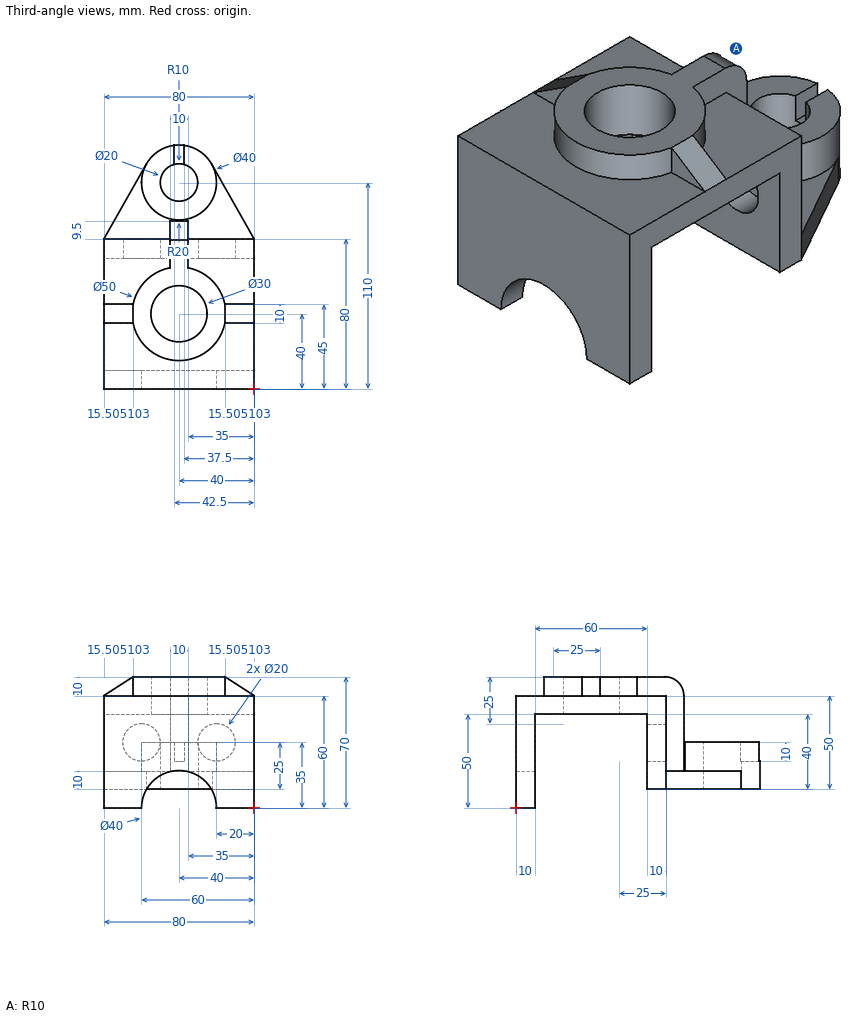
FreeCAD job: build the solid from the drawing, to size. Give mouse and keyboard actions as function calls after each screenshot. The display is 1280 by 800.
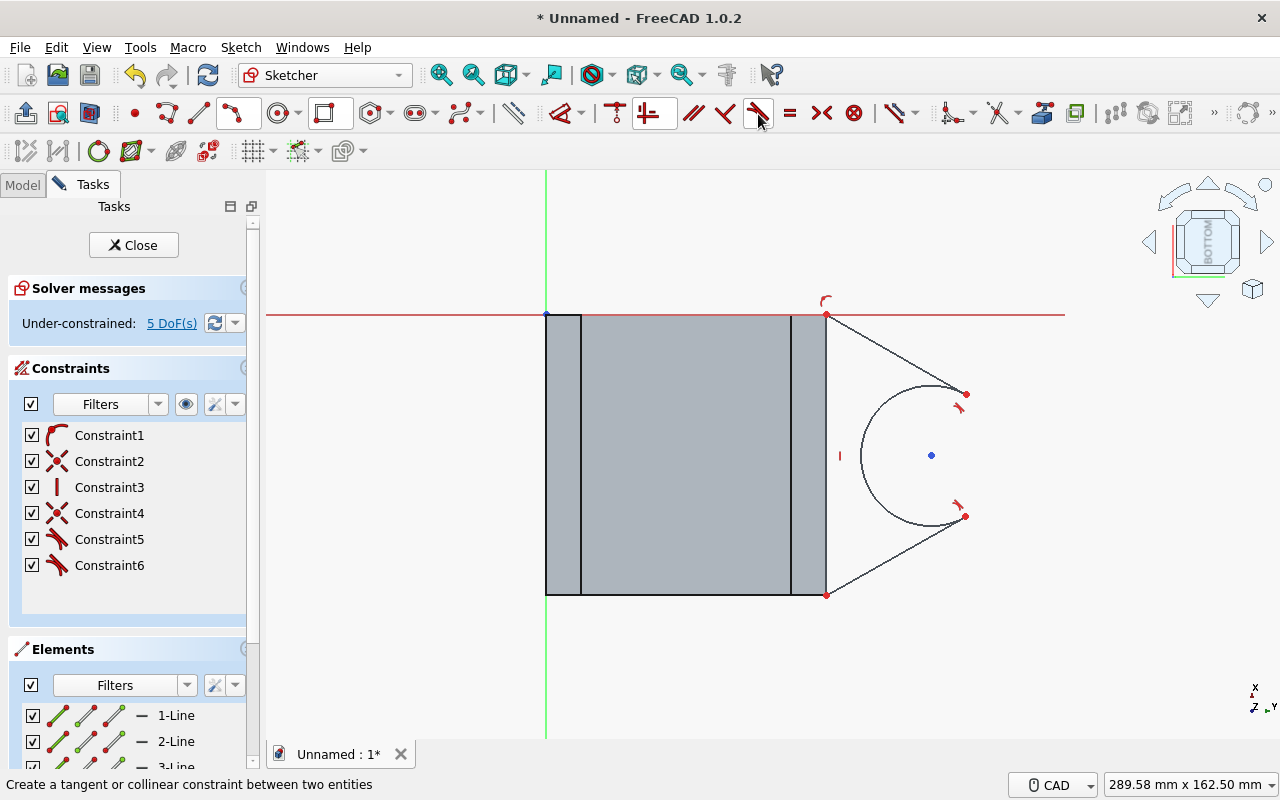
click(560, 114)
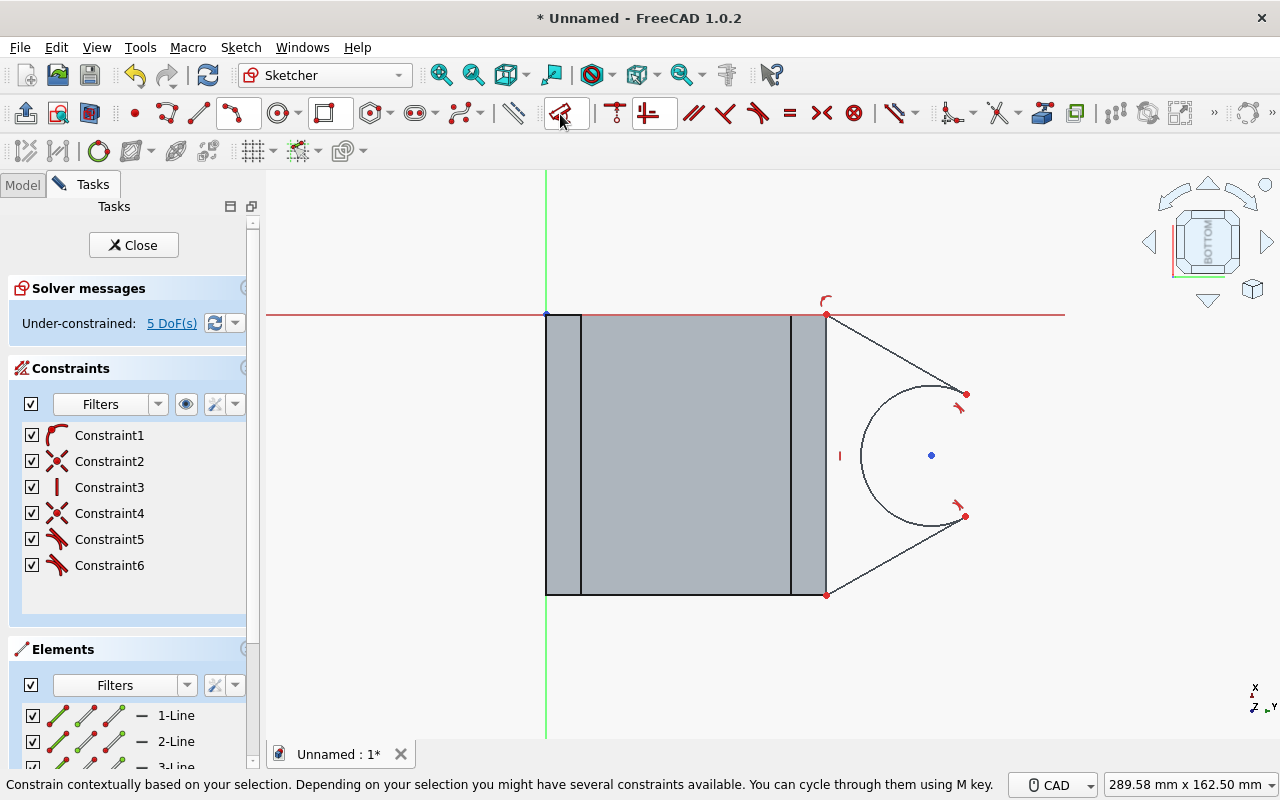
click(884, 404)
click(862, 380)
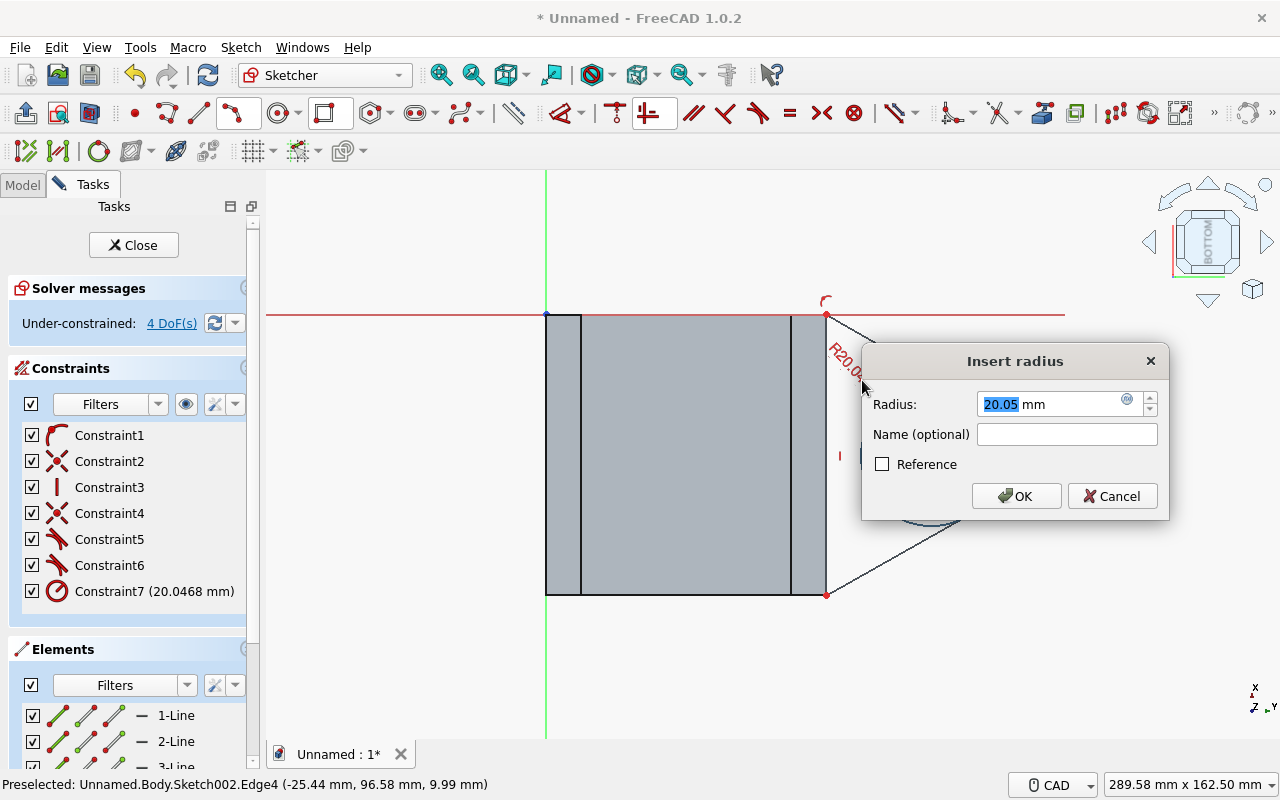
text(20)
key(Return)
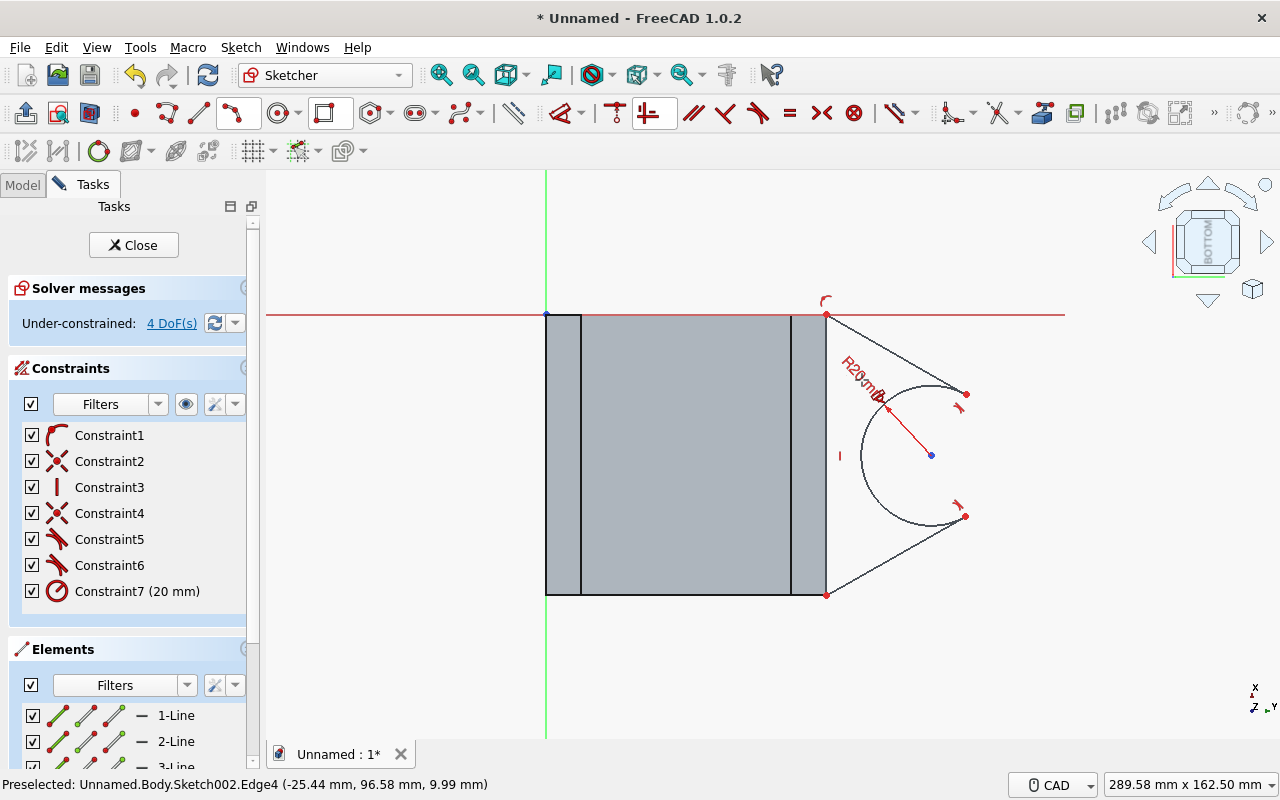
click(826, 399)
click(860, 520)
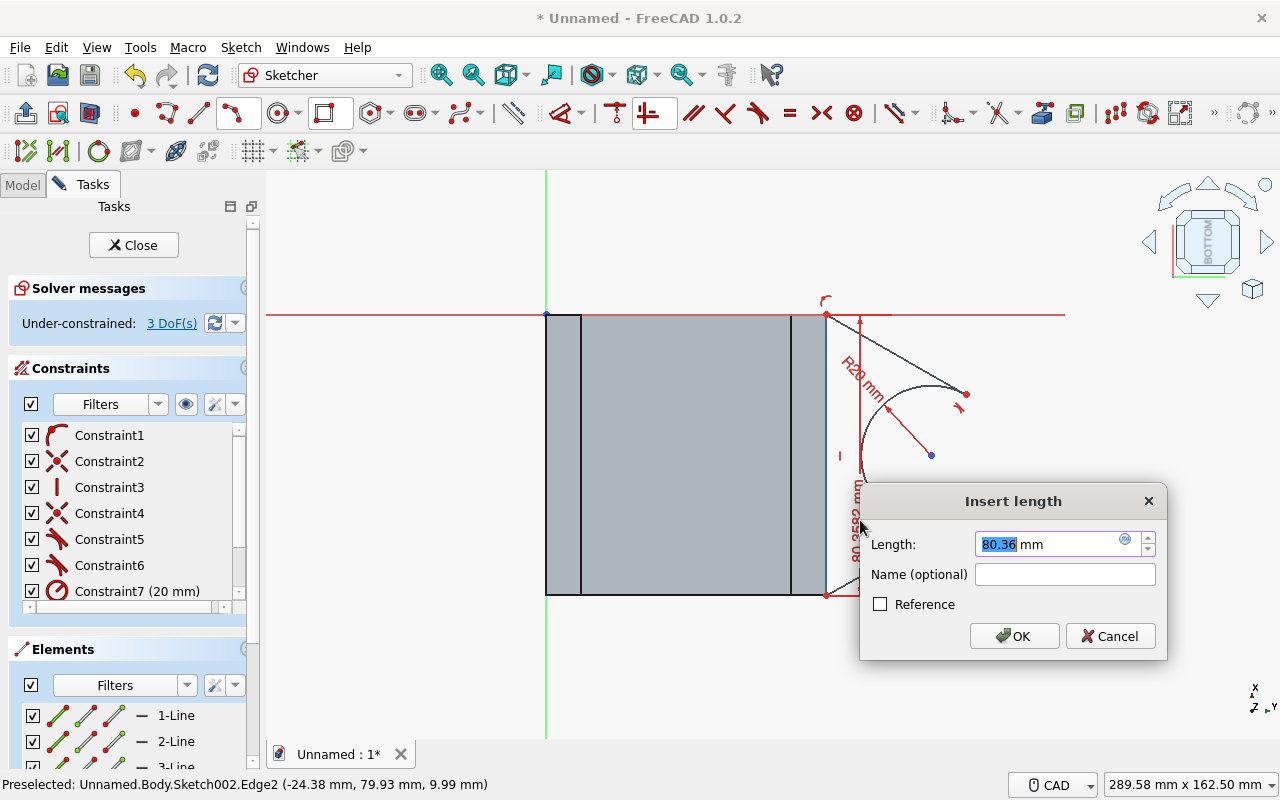
text(80)
key(Return)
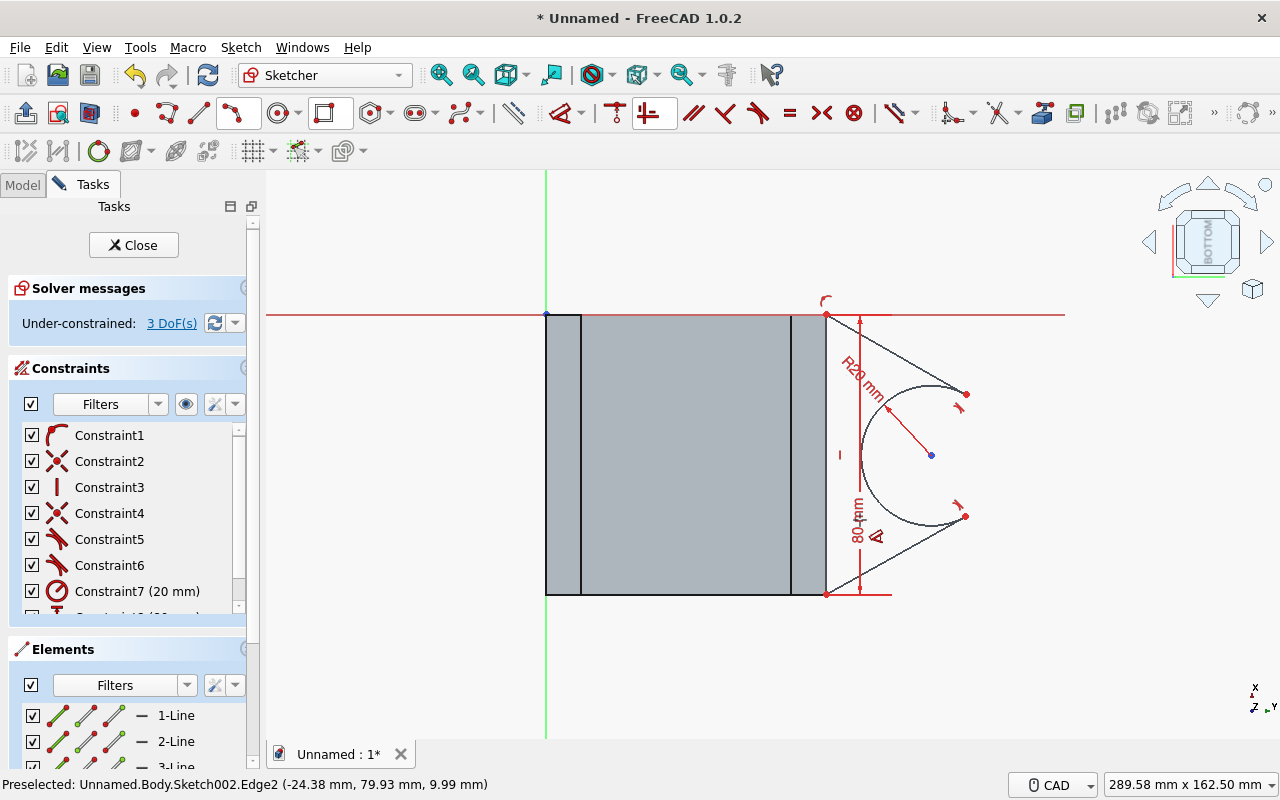
click(826, 315)
click(686, 281)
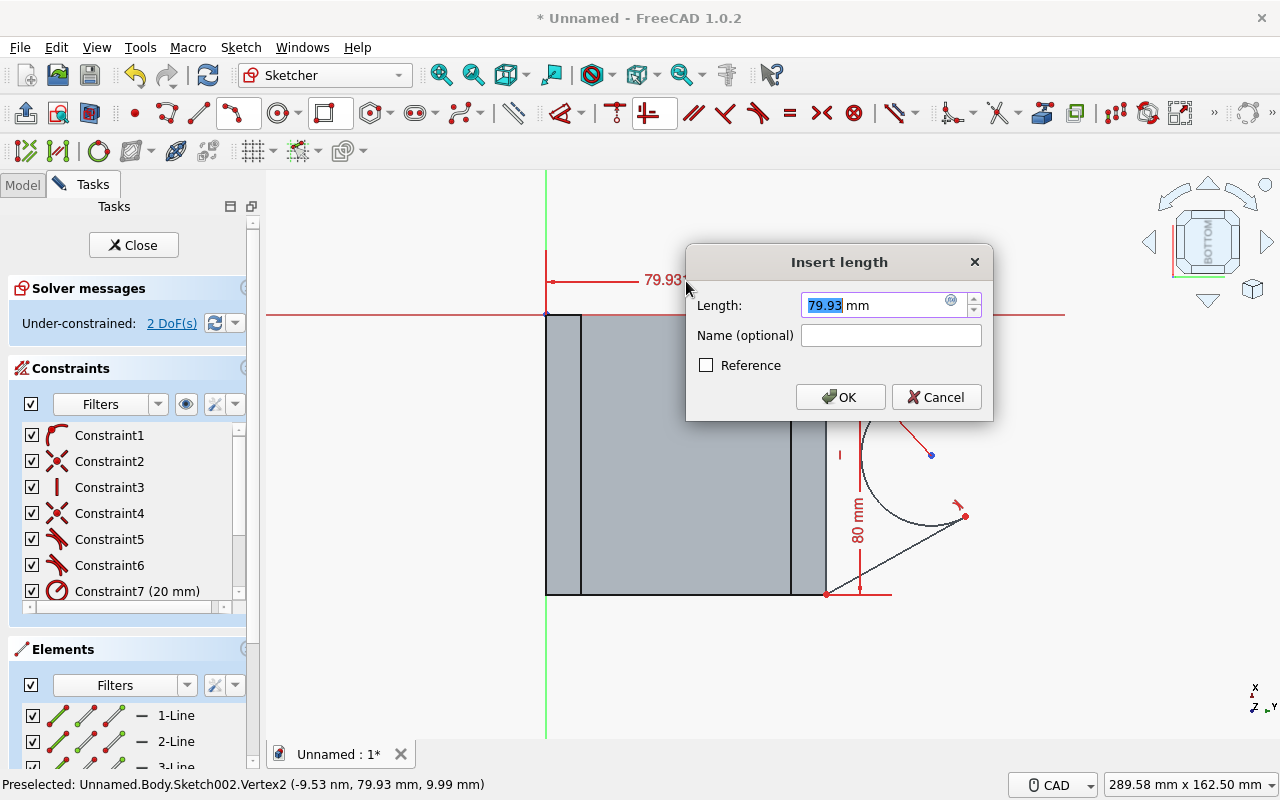
text(80)
key(Return)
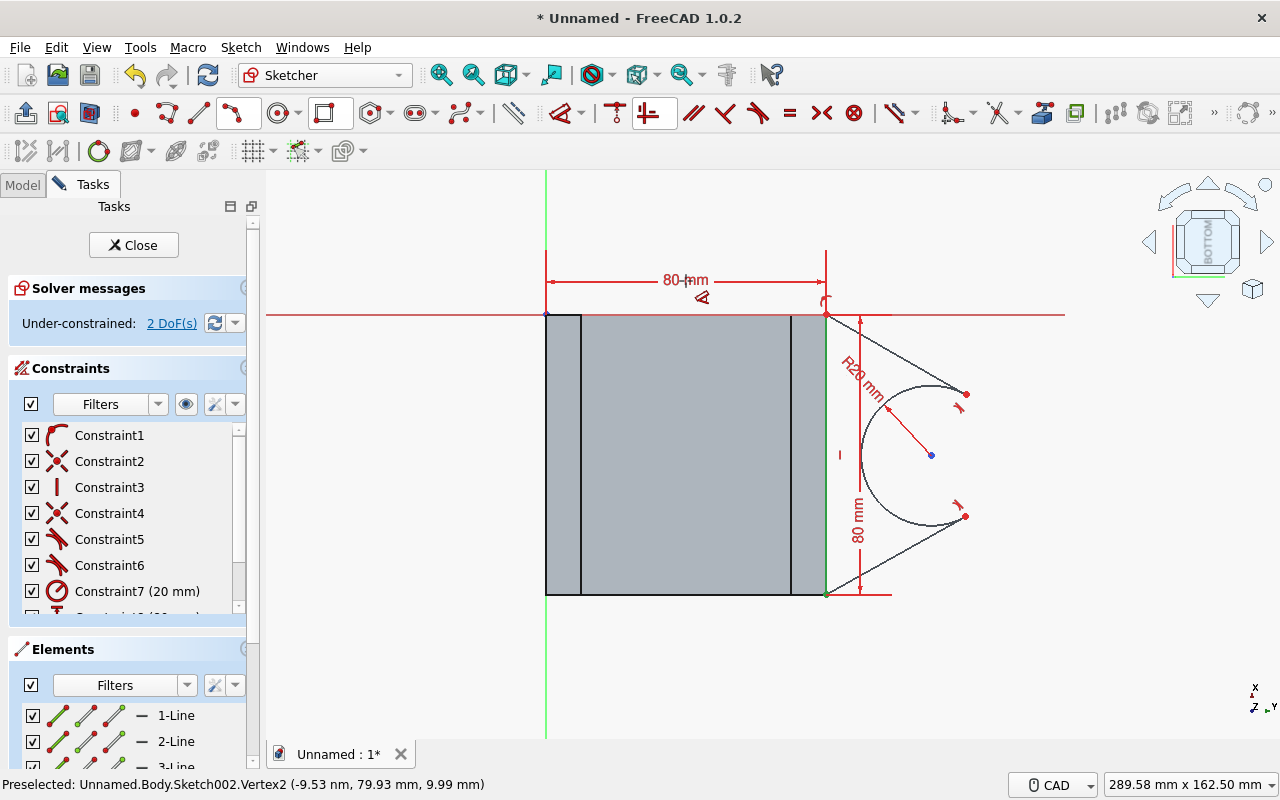
click(931, 456)
click(512, 385)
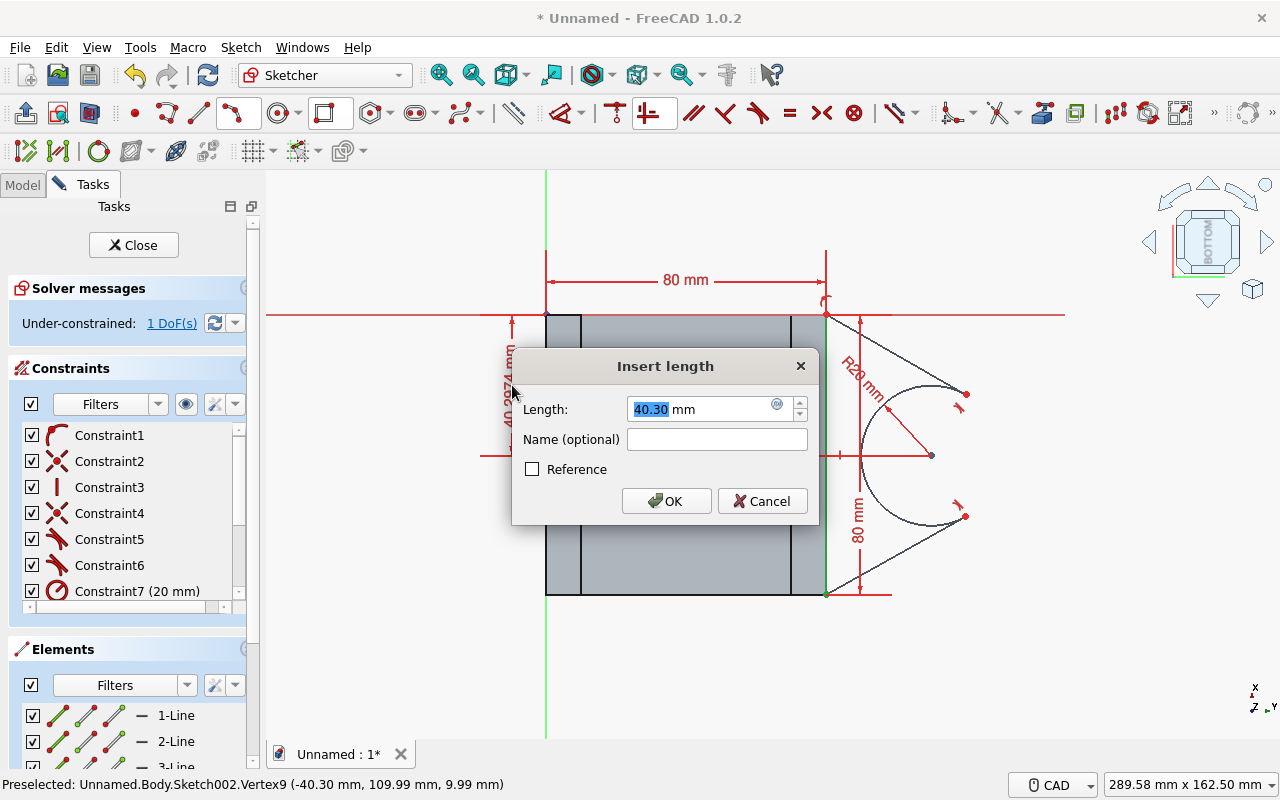
text(40)
key(Return)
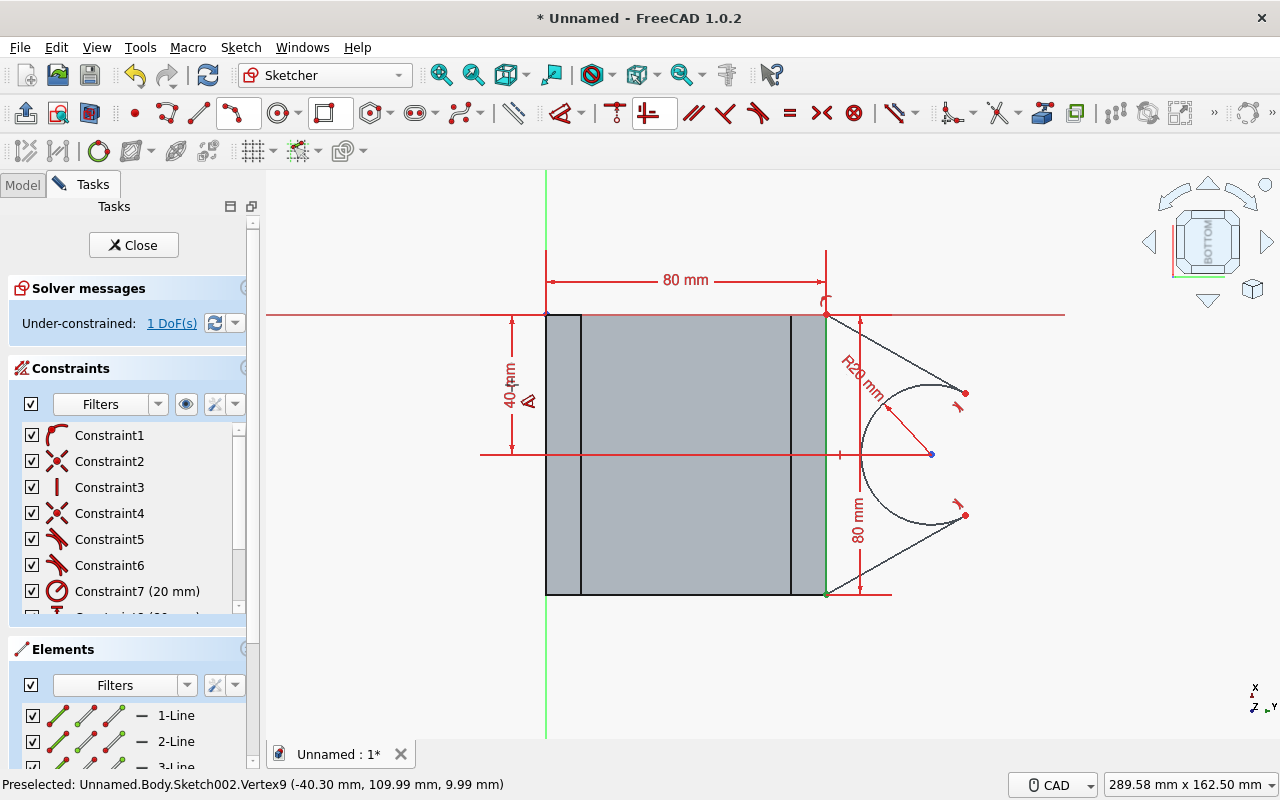
click(931, 455)
click(827, 281)